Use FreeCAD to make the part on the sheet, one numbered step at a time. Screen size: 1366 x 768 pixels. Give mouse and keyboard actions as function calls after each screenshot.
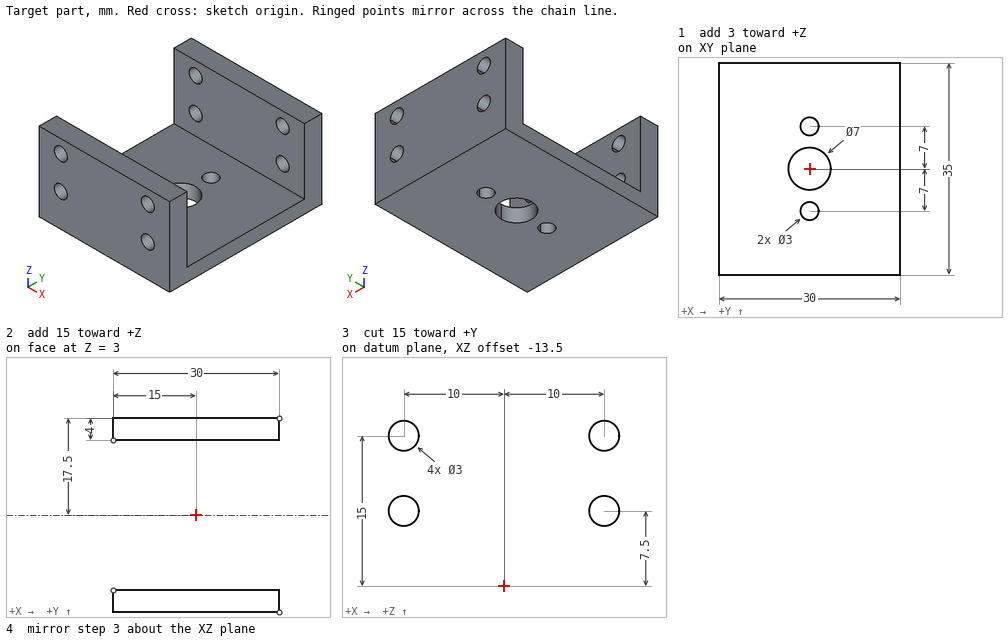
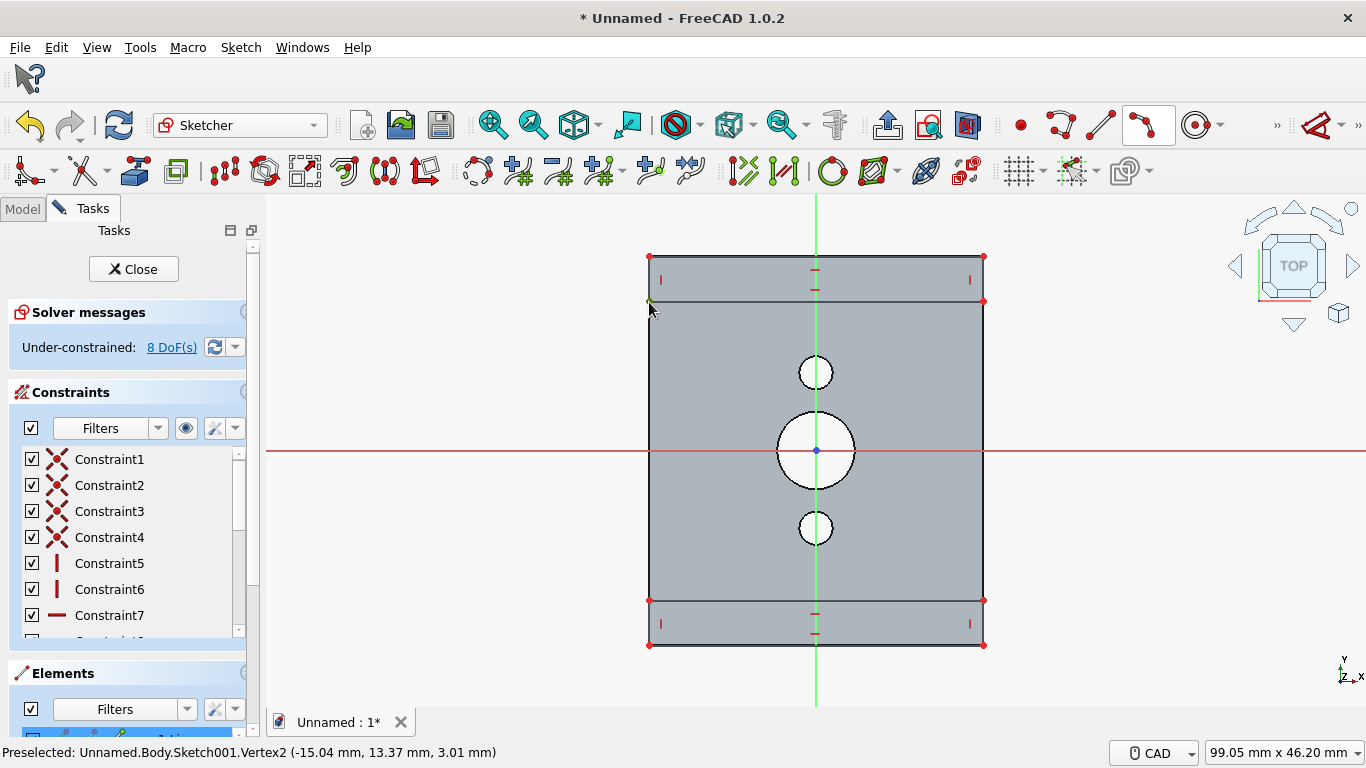
click(649, 601)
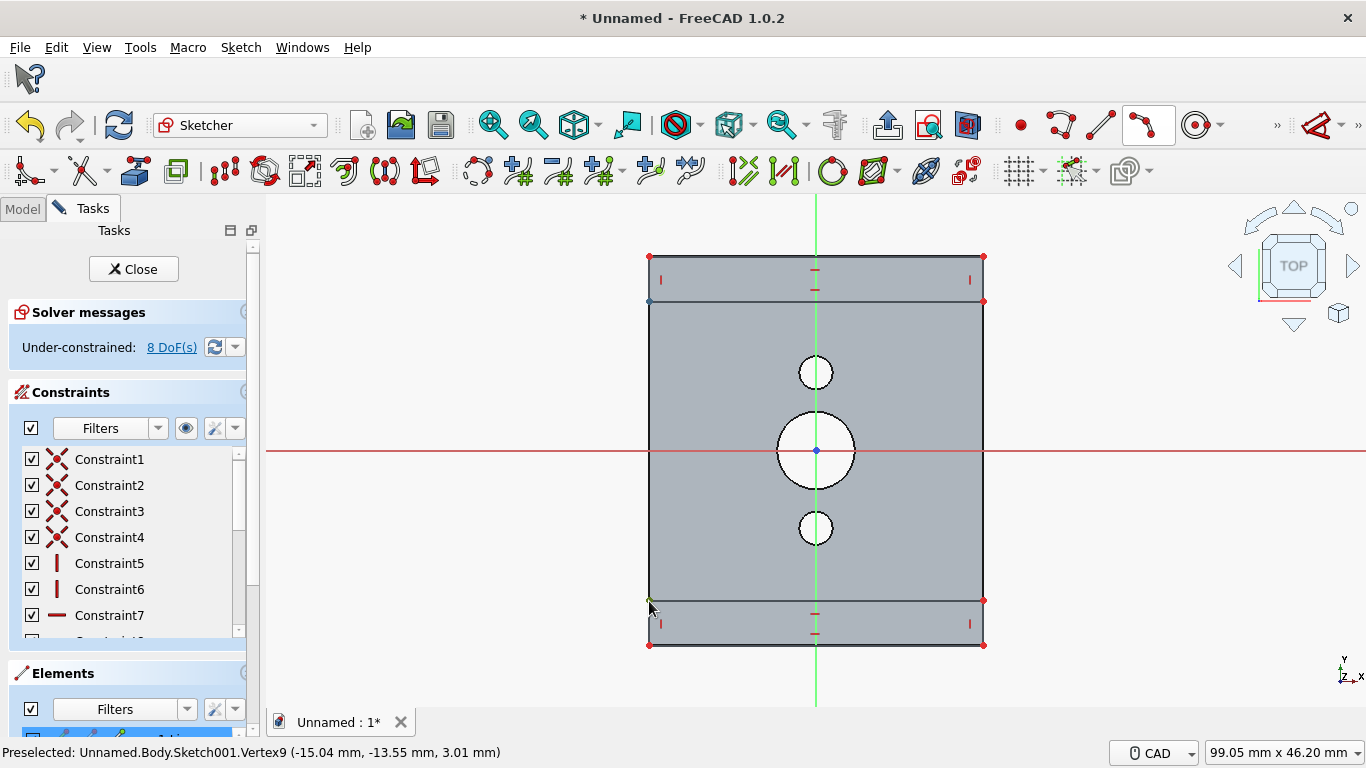
click(359, 450)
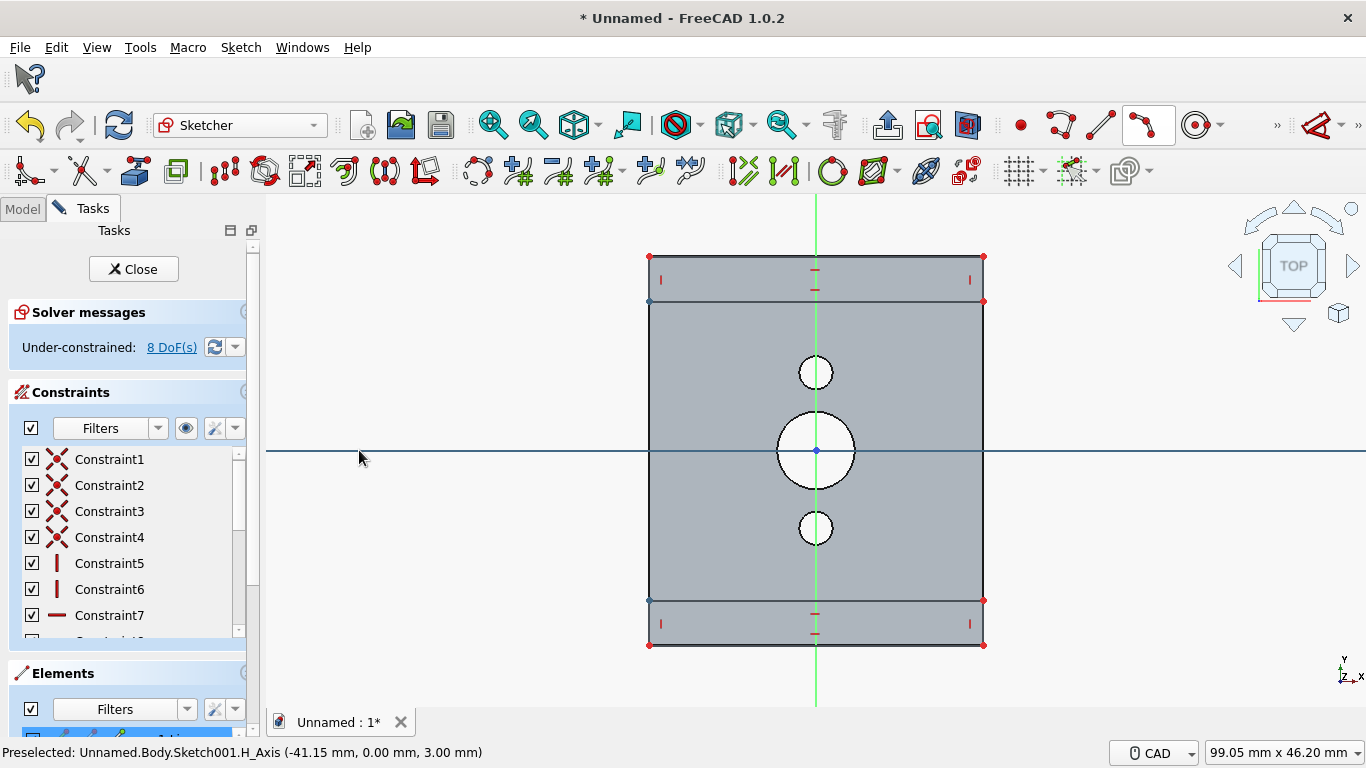
key(s)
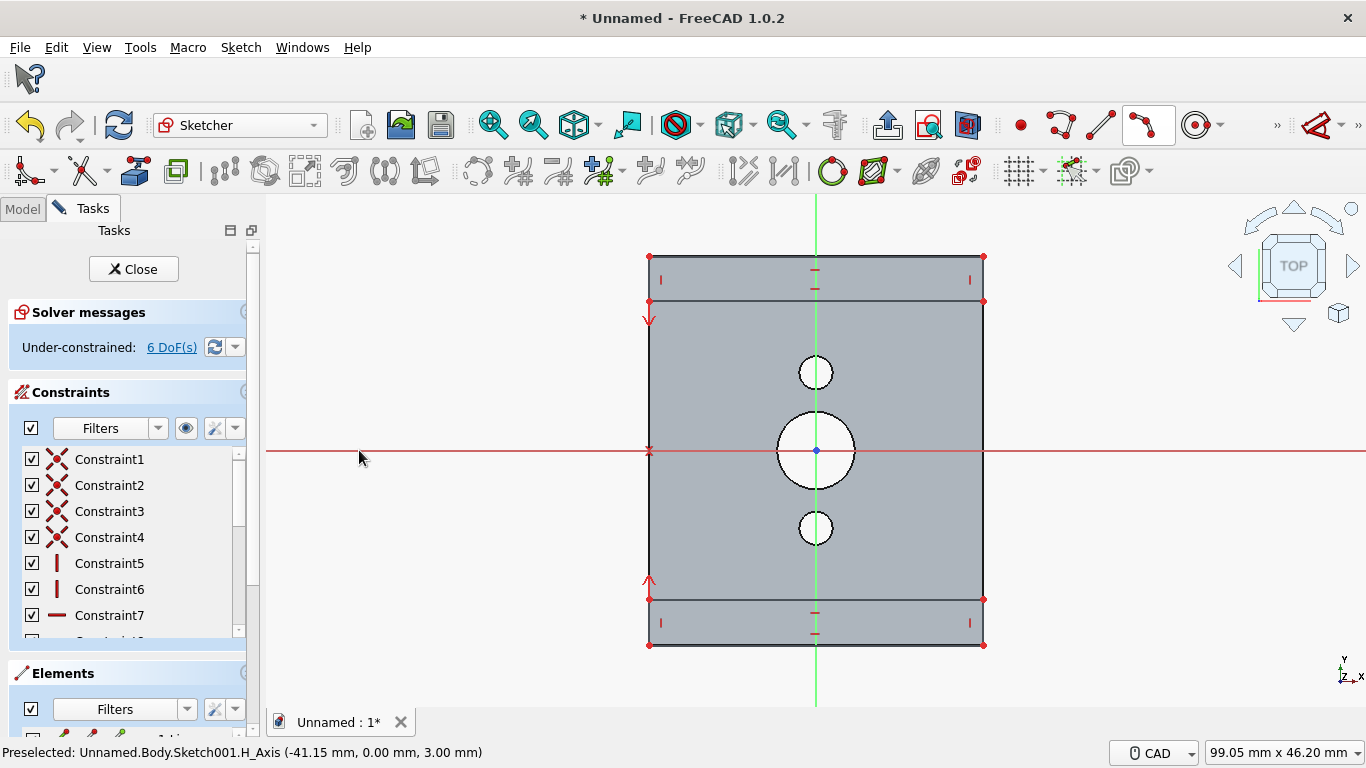
click(983, 257)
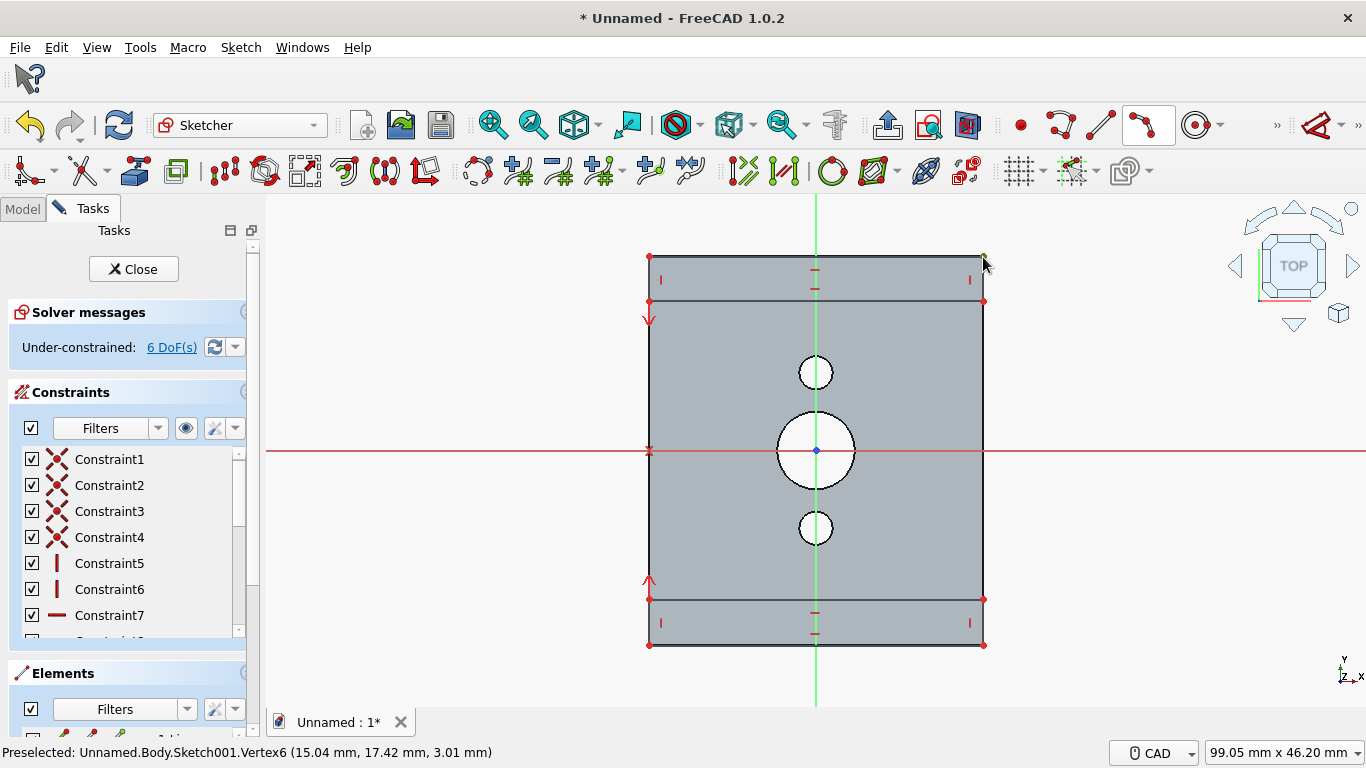
click(983, 646)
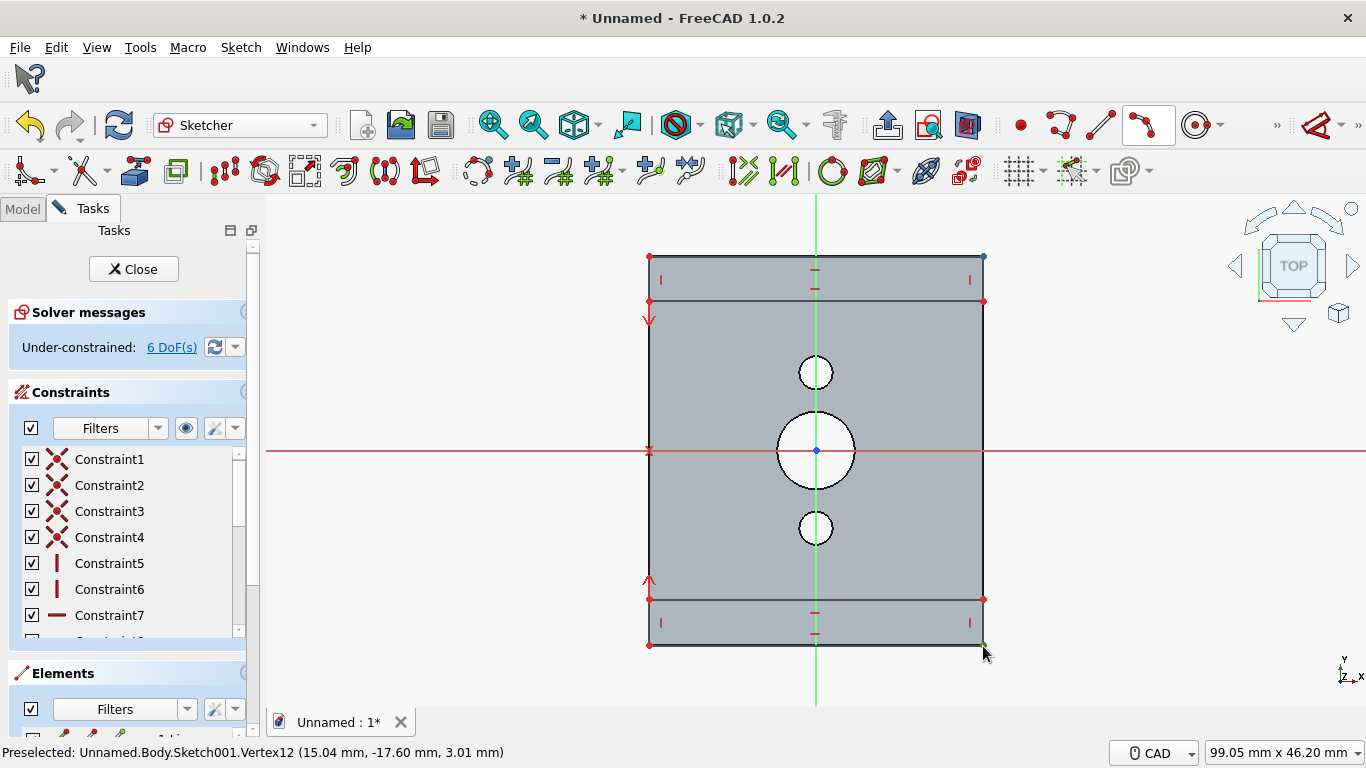
click(359, 450)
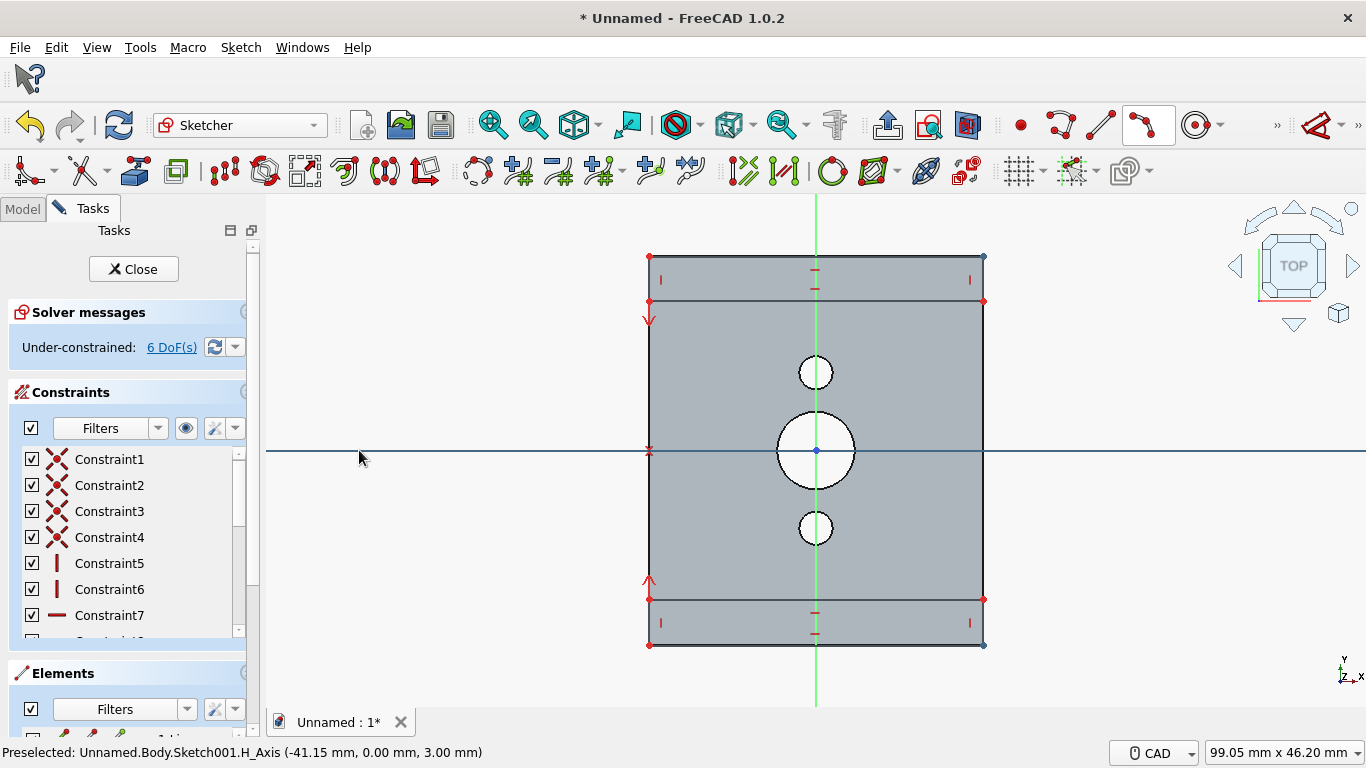
key(s)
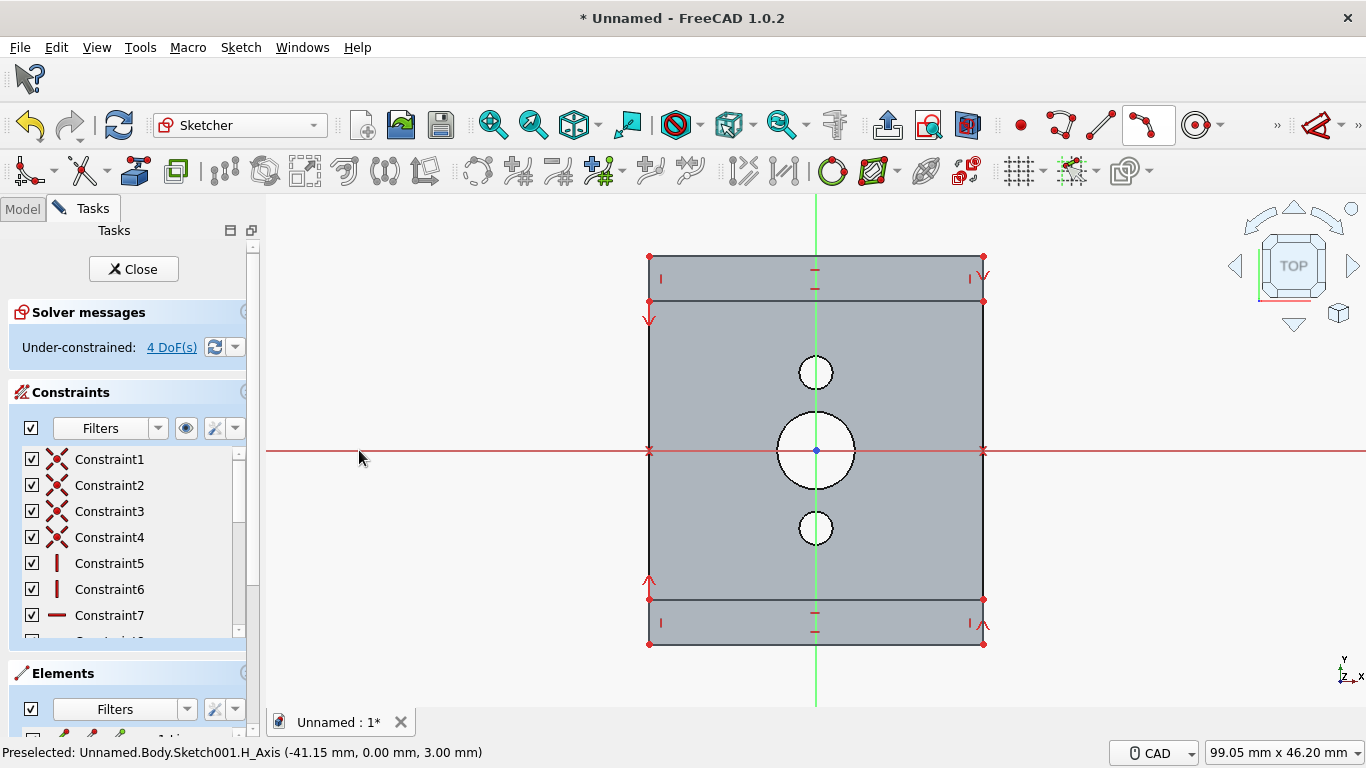
key(d)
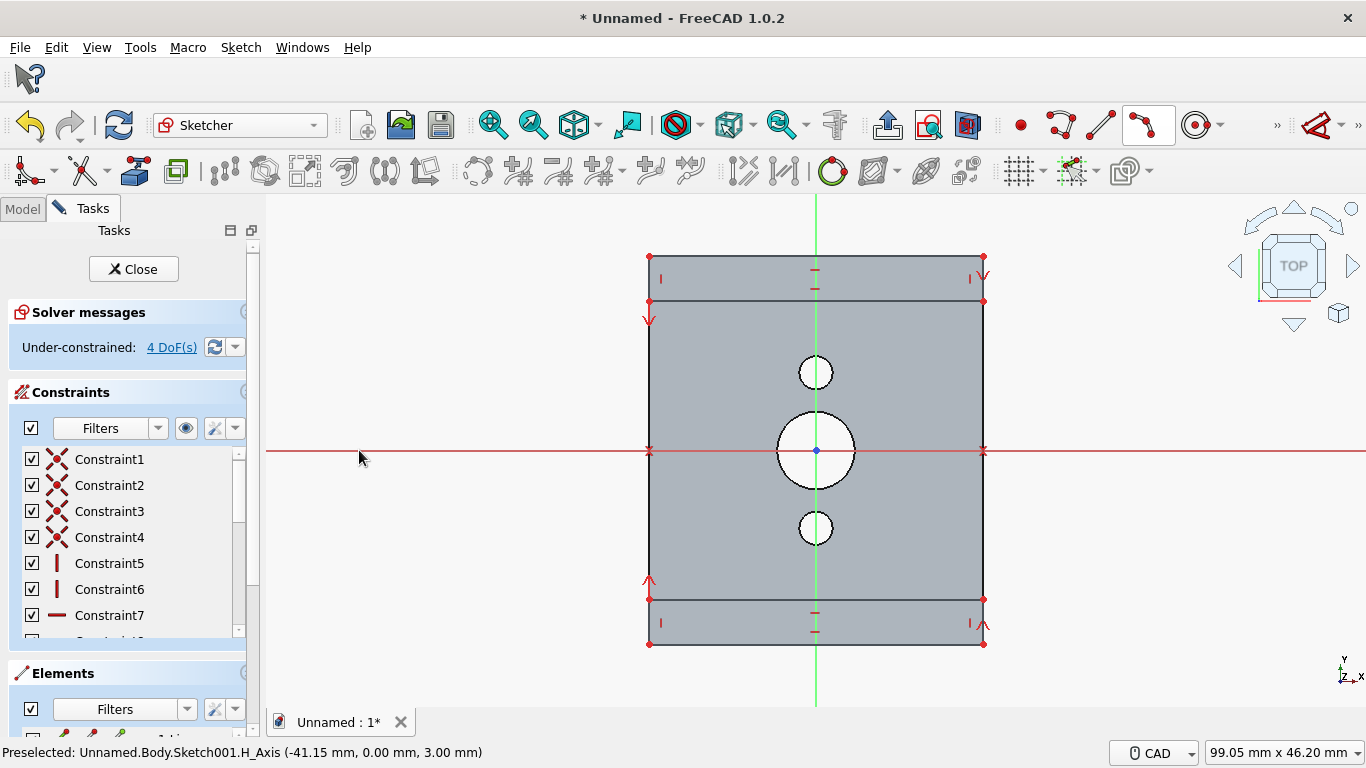
click(649, 270)
click(615, 279)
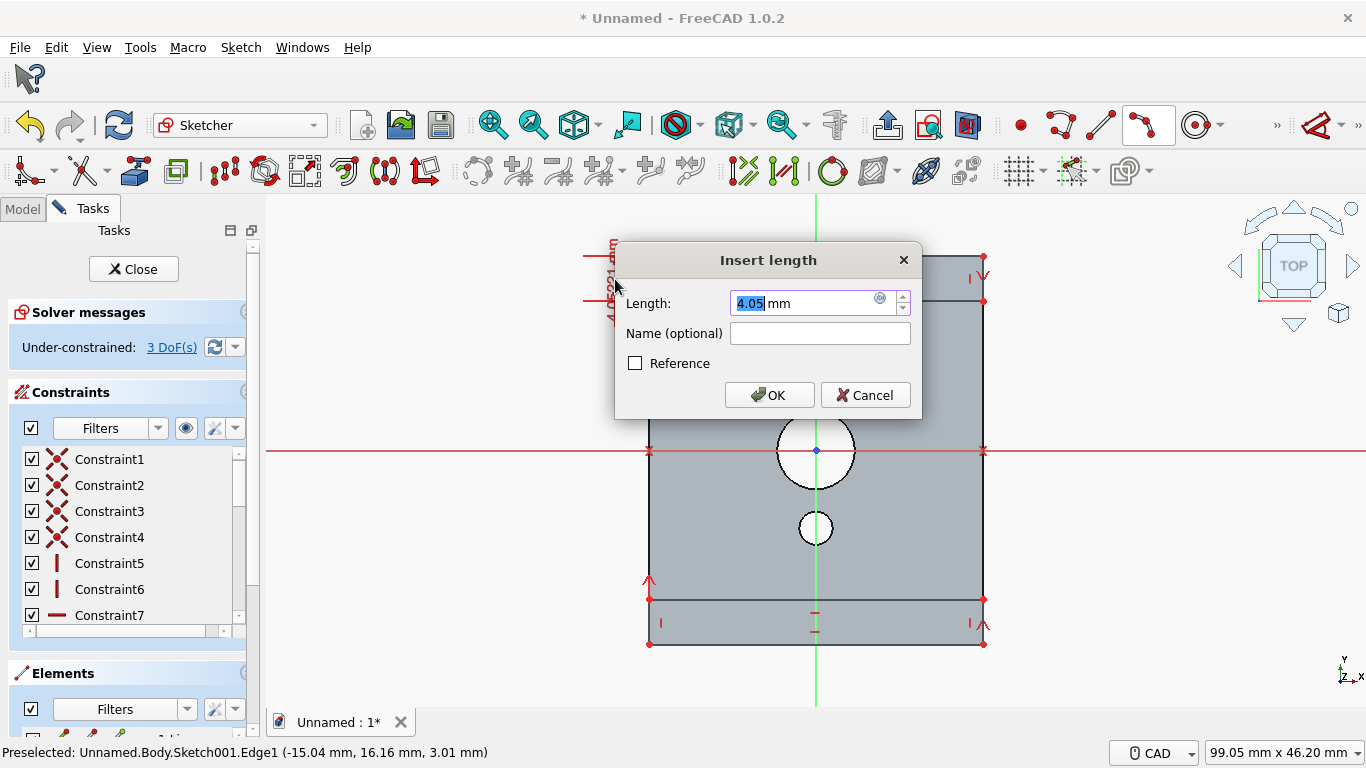
text(4)
key(Return)